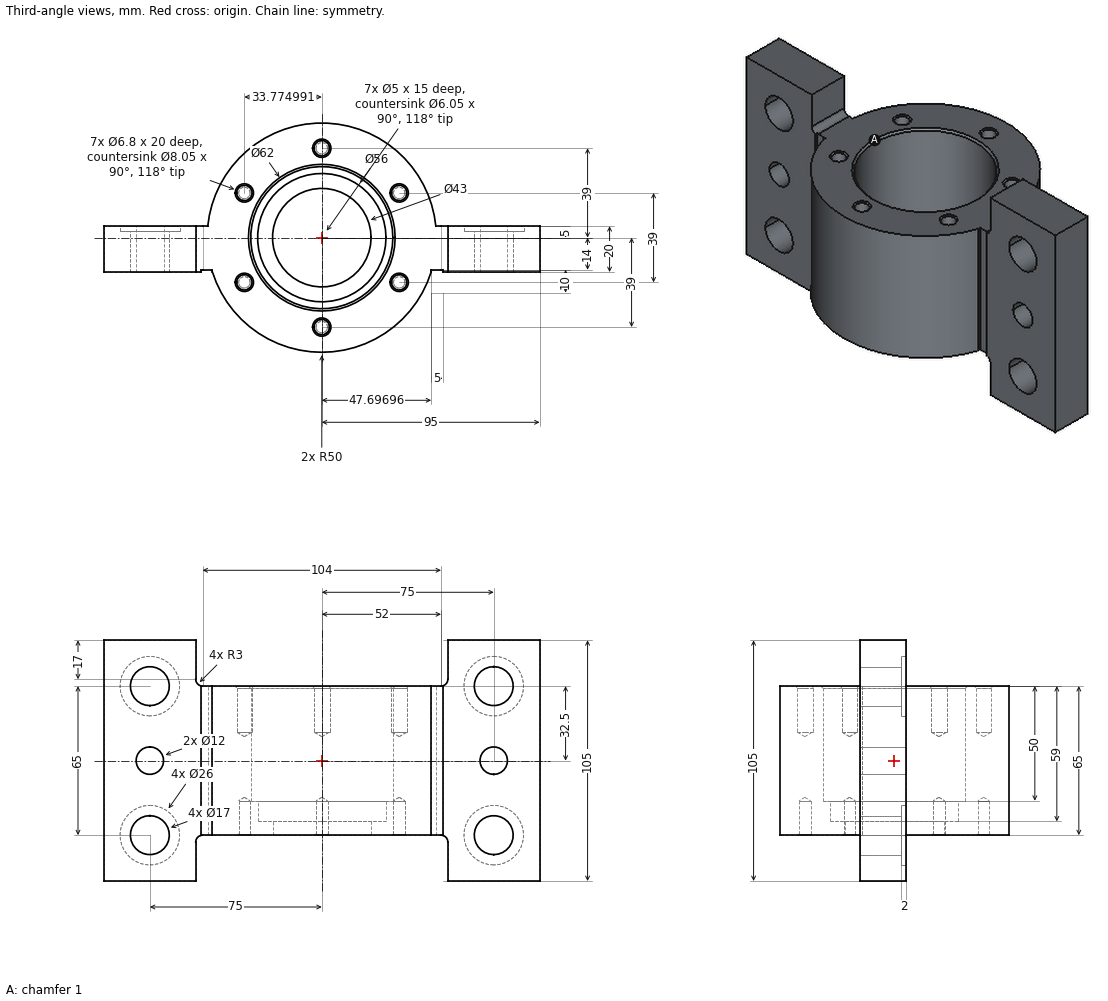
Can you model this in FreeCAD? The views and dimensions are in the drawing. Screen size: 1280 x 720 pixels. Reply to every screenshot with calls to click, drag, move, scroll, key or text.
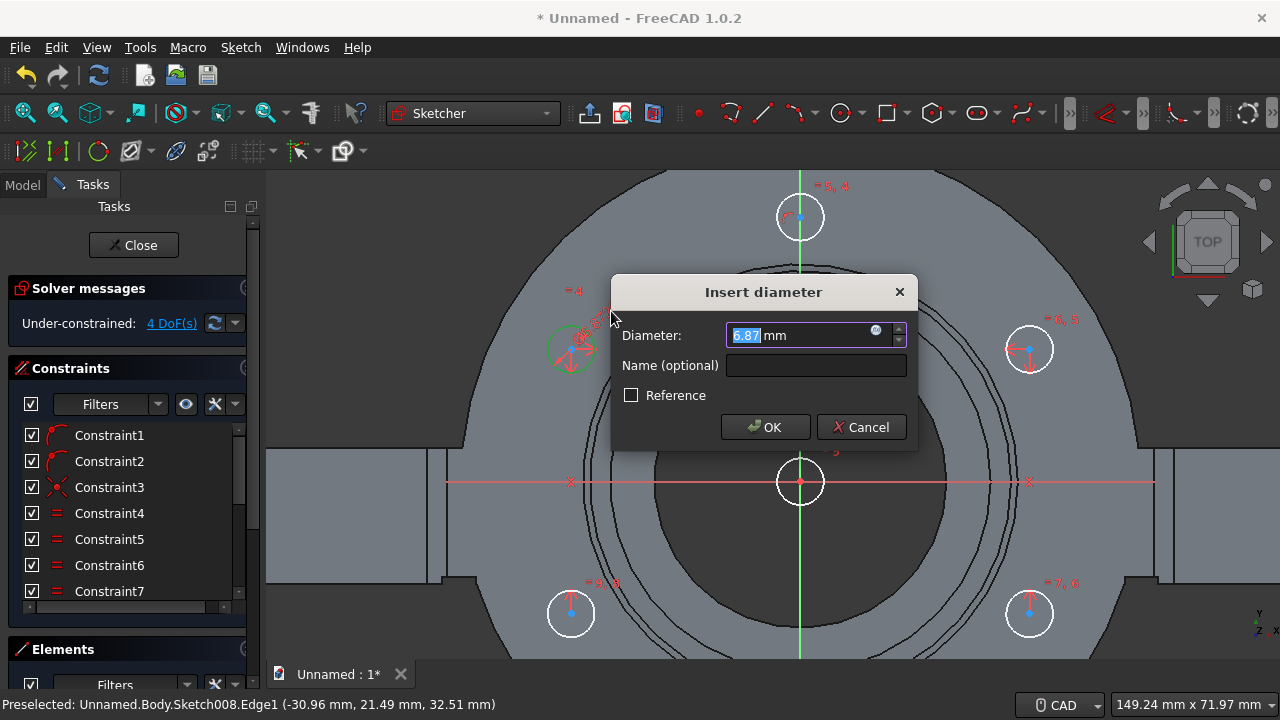
text(6.8)
key(Return)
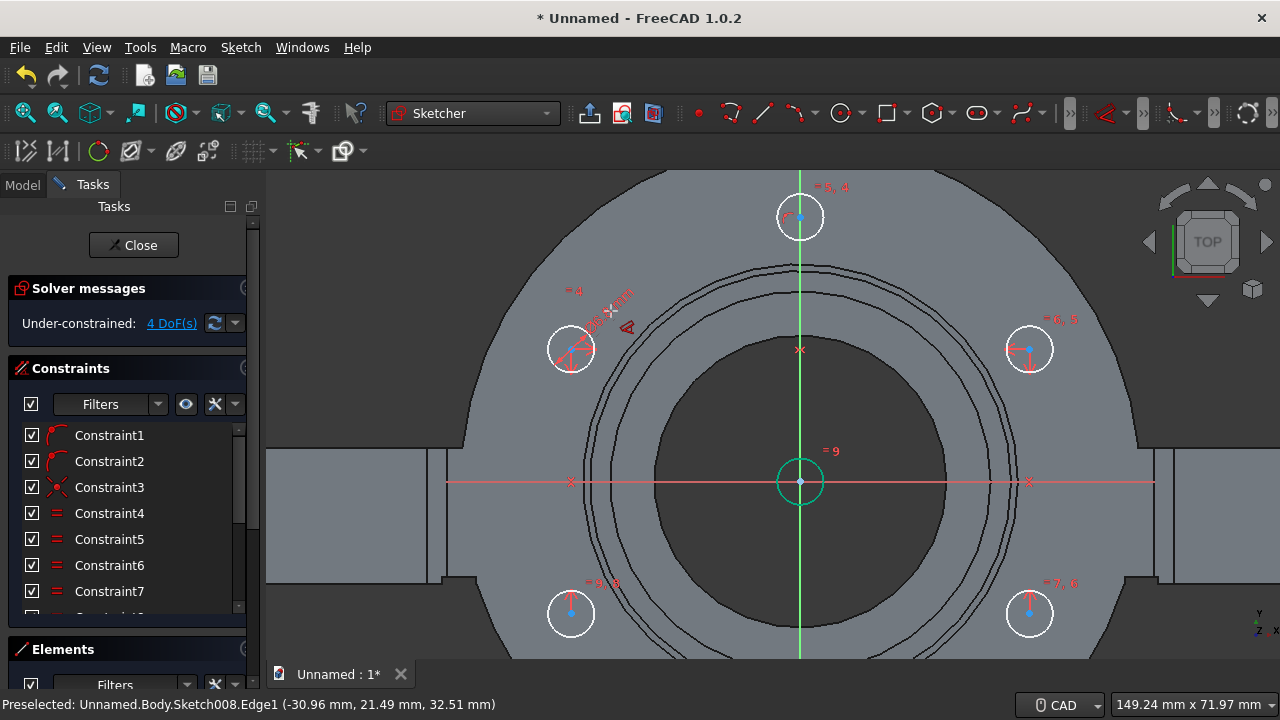
click(800, 217)
click(834, 349)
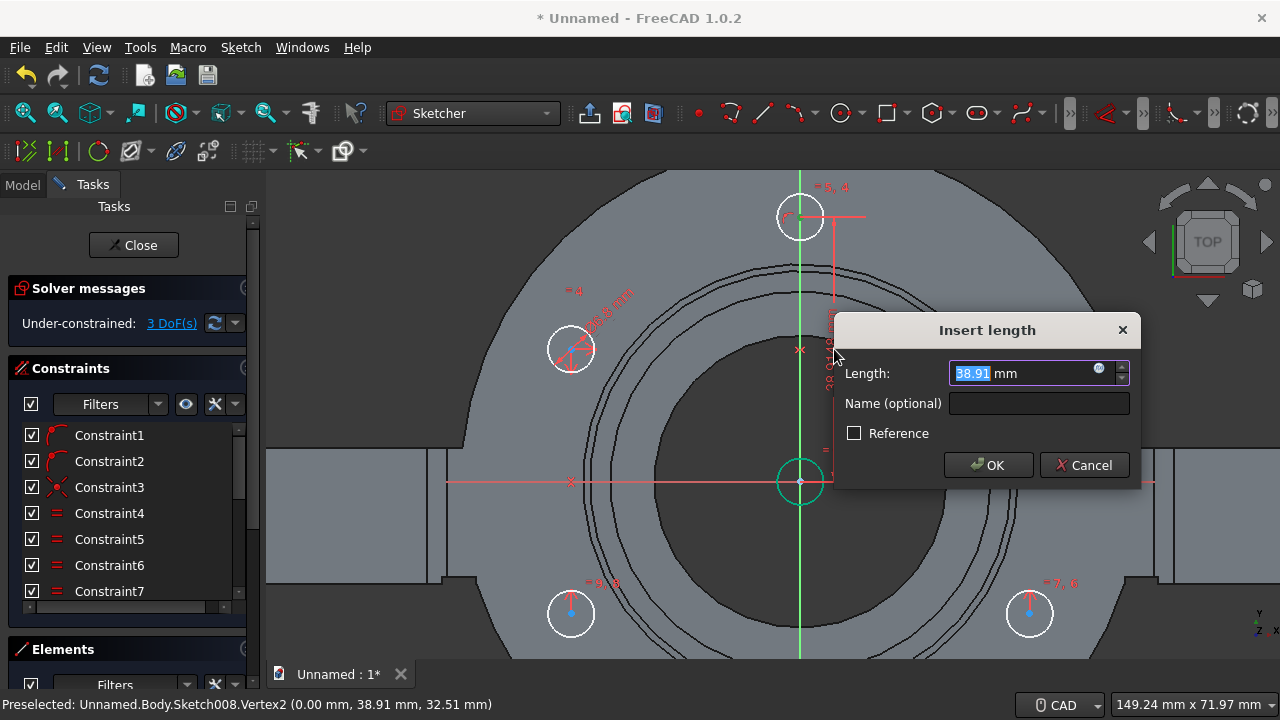
text(39)
key(Return)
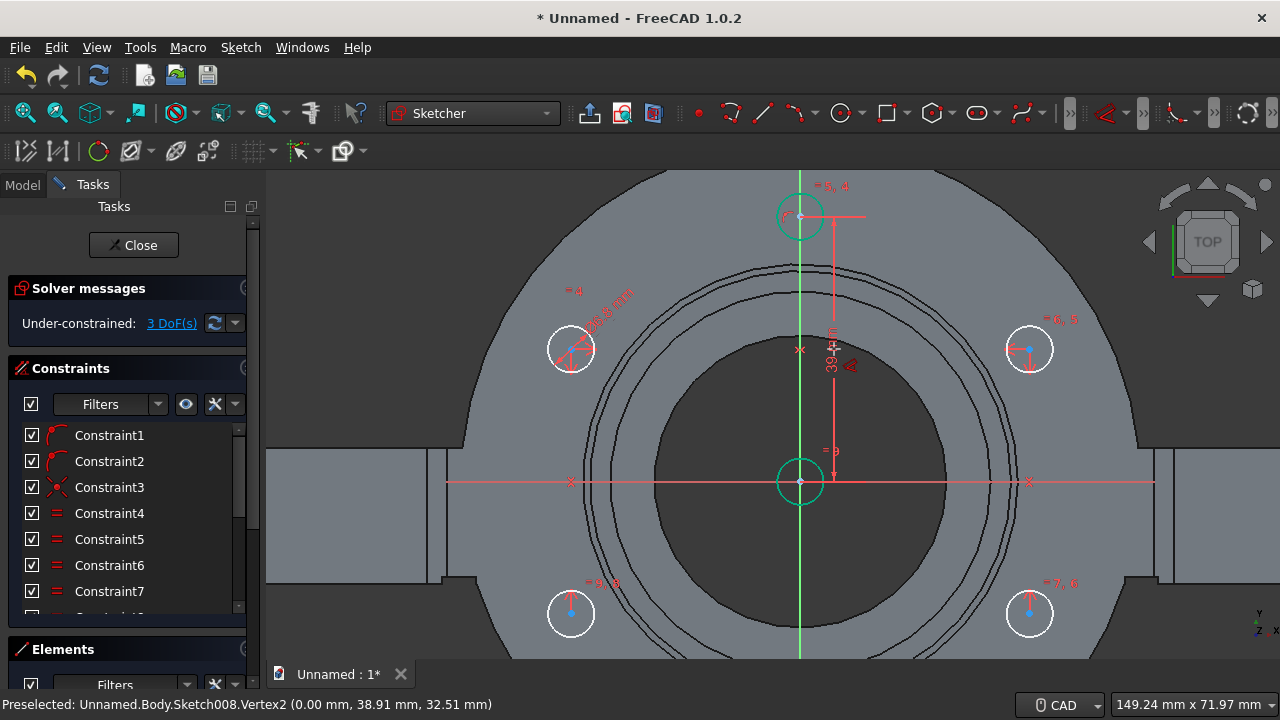
scroll(588, 333, down, 3)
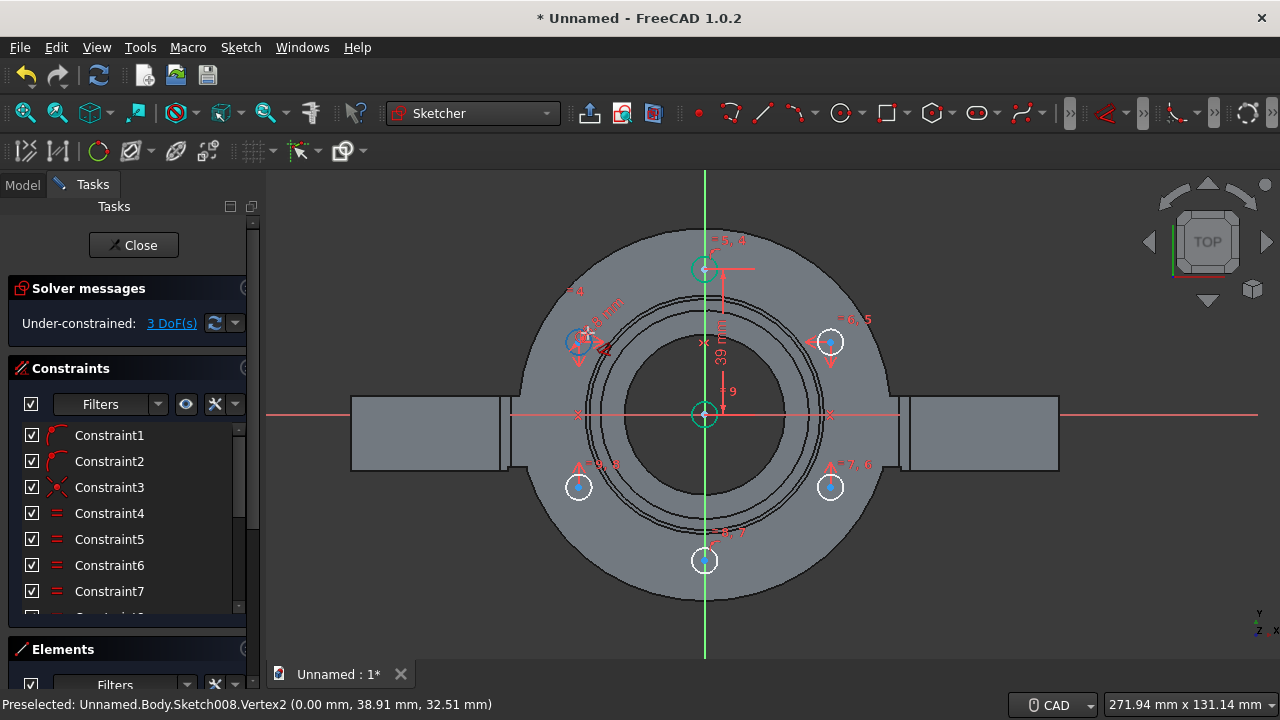
click(705, 561)
click(739, 488)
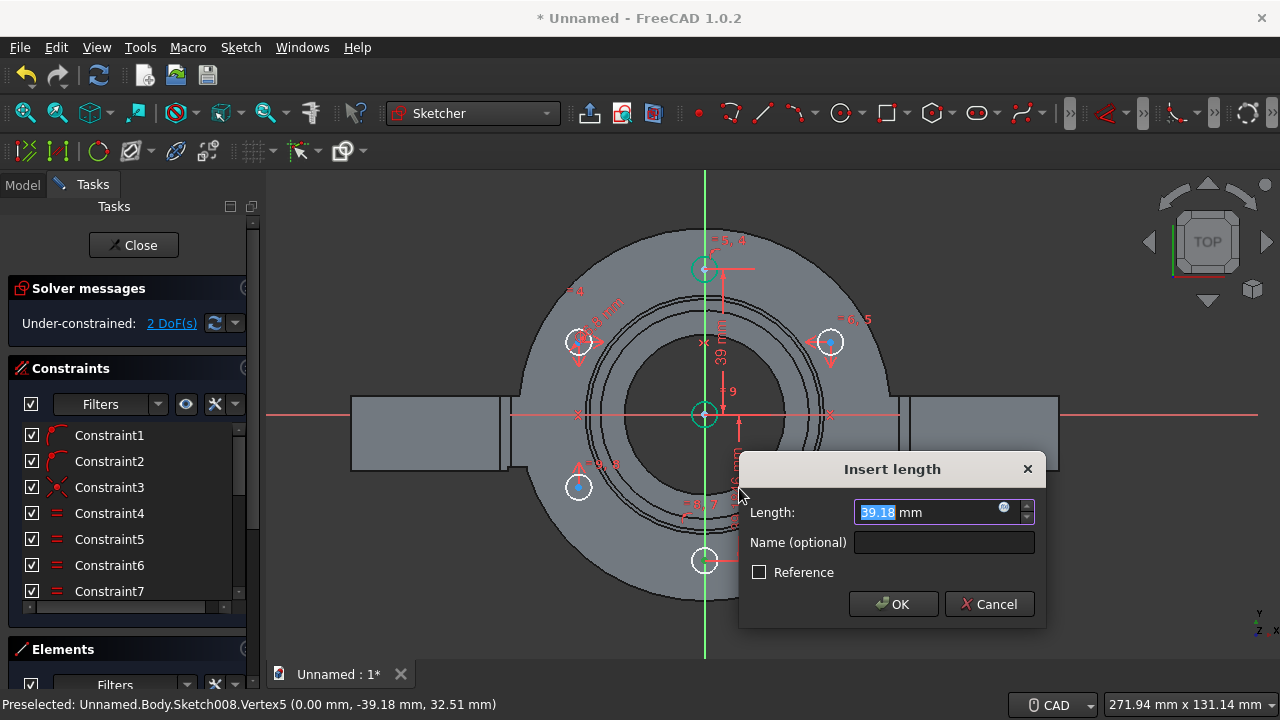
text(39)
key(Return)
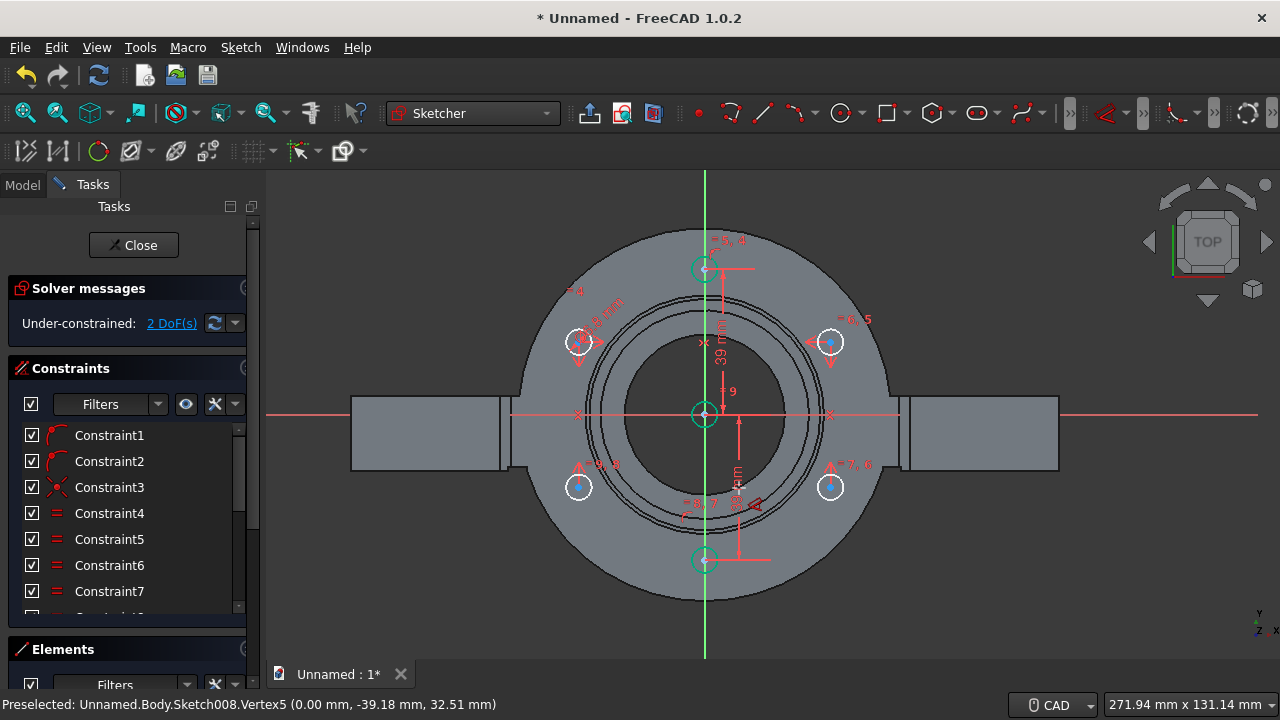
click(831, 342)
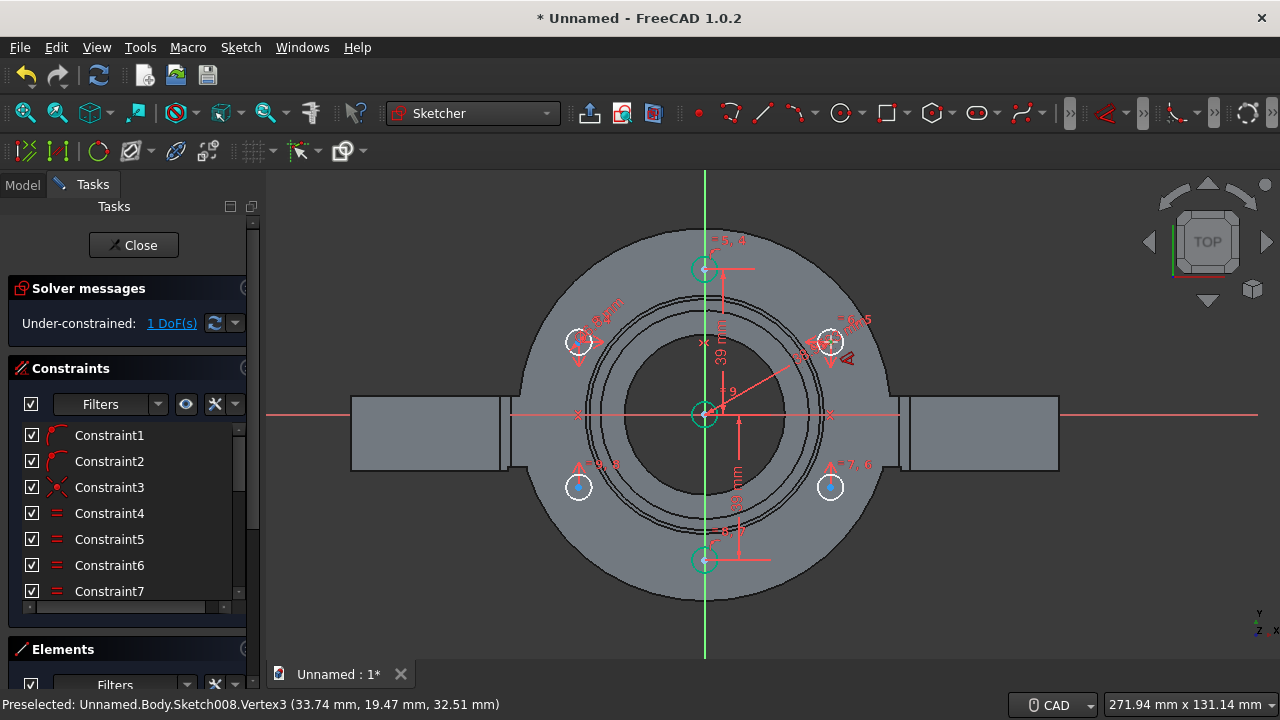
click(831, 487)
click(865, 381)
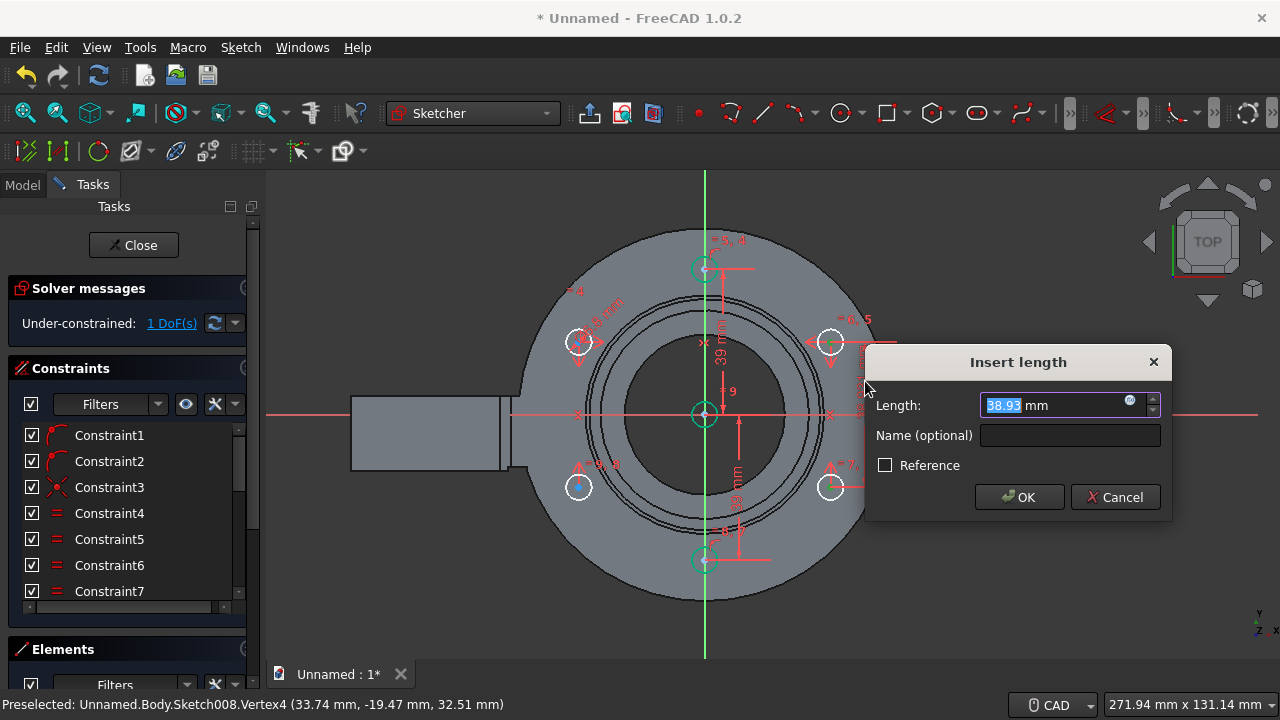
text(39)
key(Return)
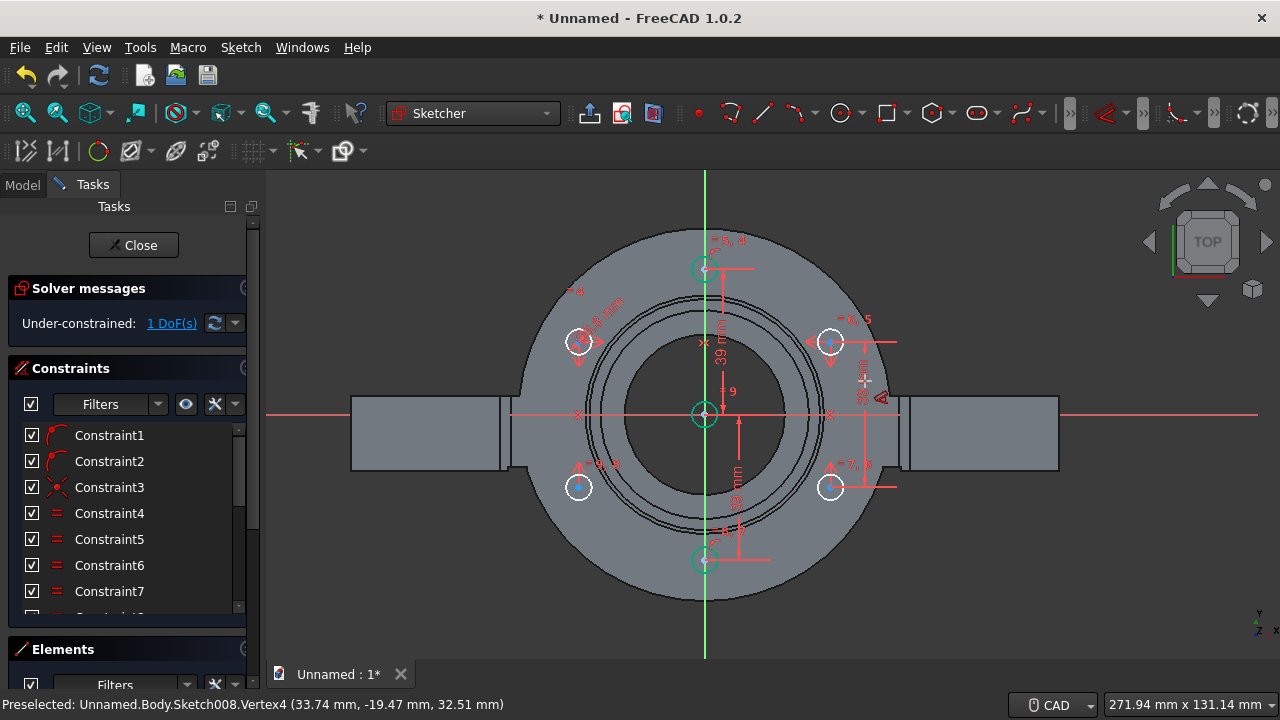
click(579, 342)
click(671, 308)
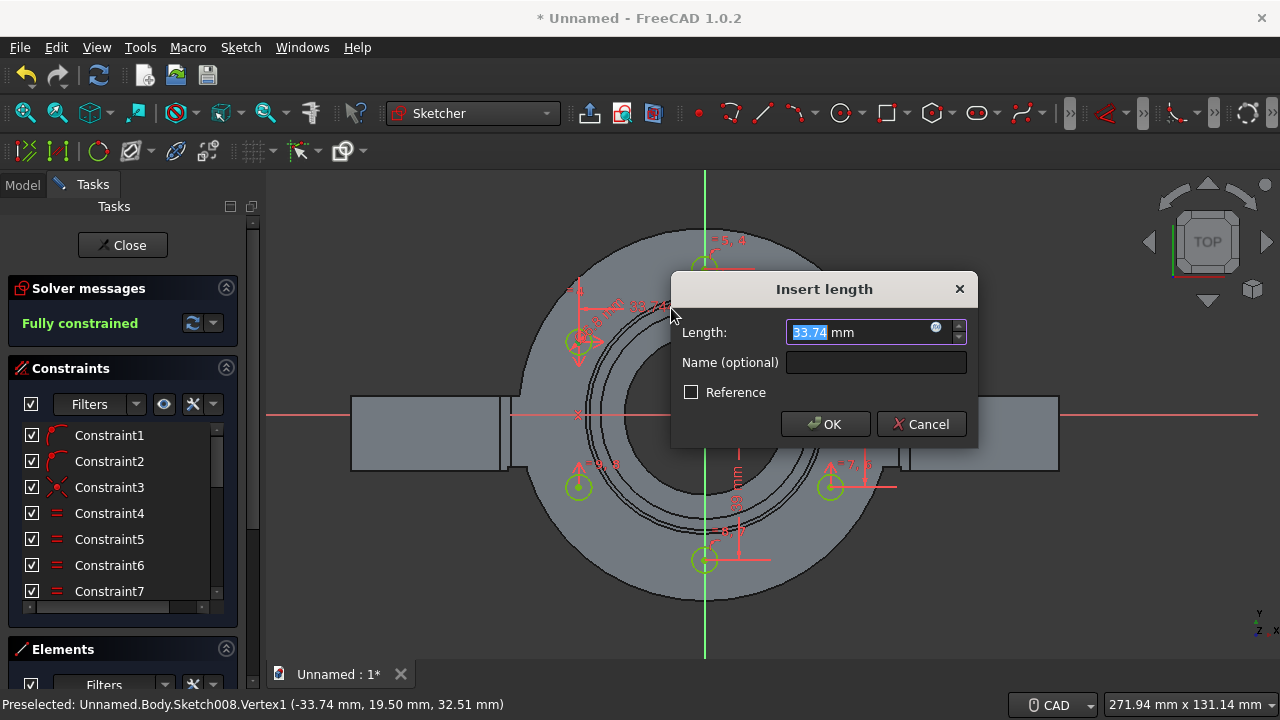
text(33.774991)
key(Return)
key(Escape)